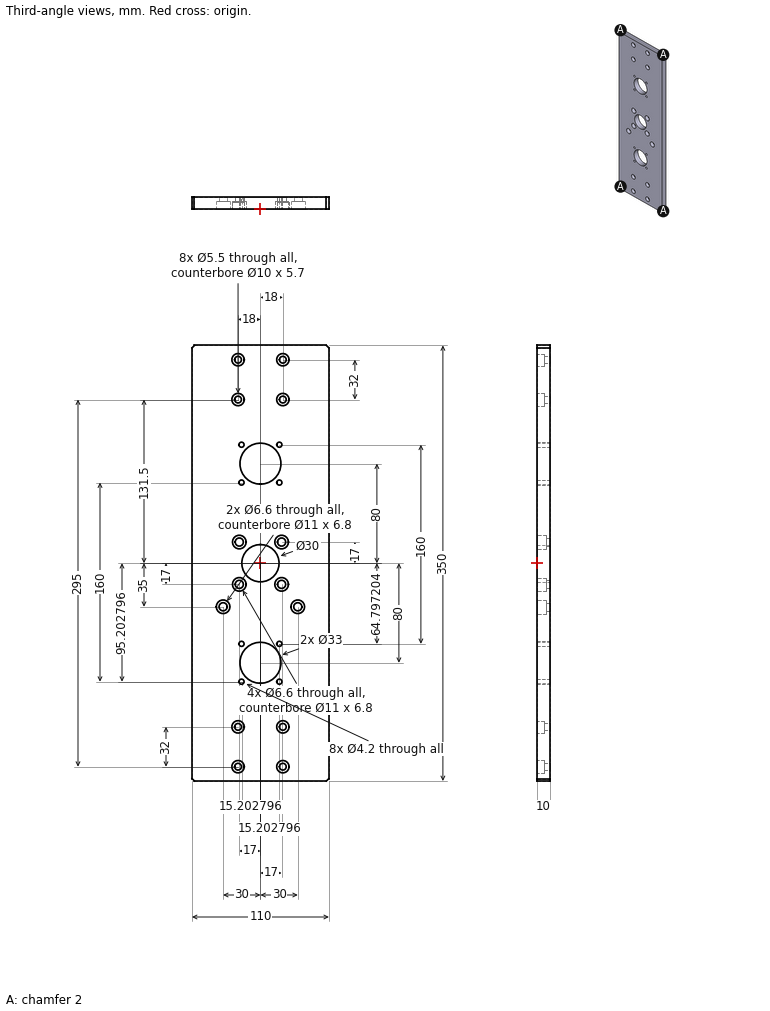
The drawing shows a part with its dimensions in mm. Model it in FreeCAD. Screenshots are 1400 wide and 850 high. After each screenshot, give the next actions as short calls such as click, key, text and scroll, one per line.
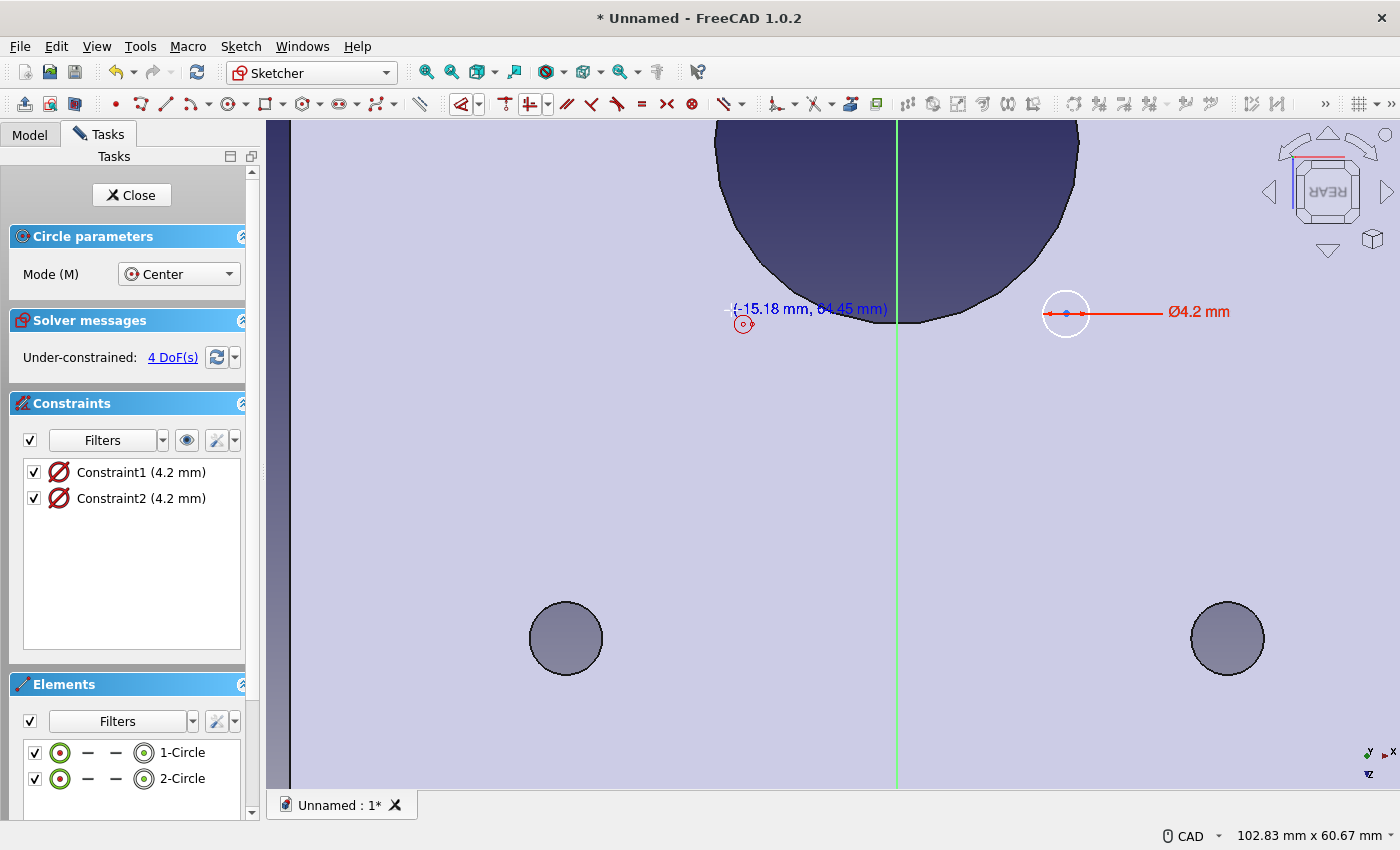
scroll(731, 310, down, 8)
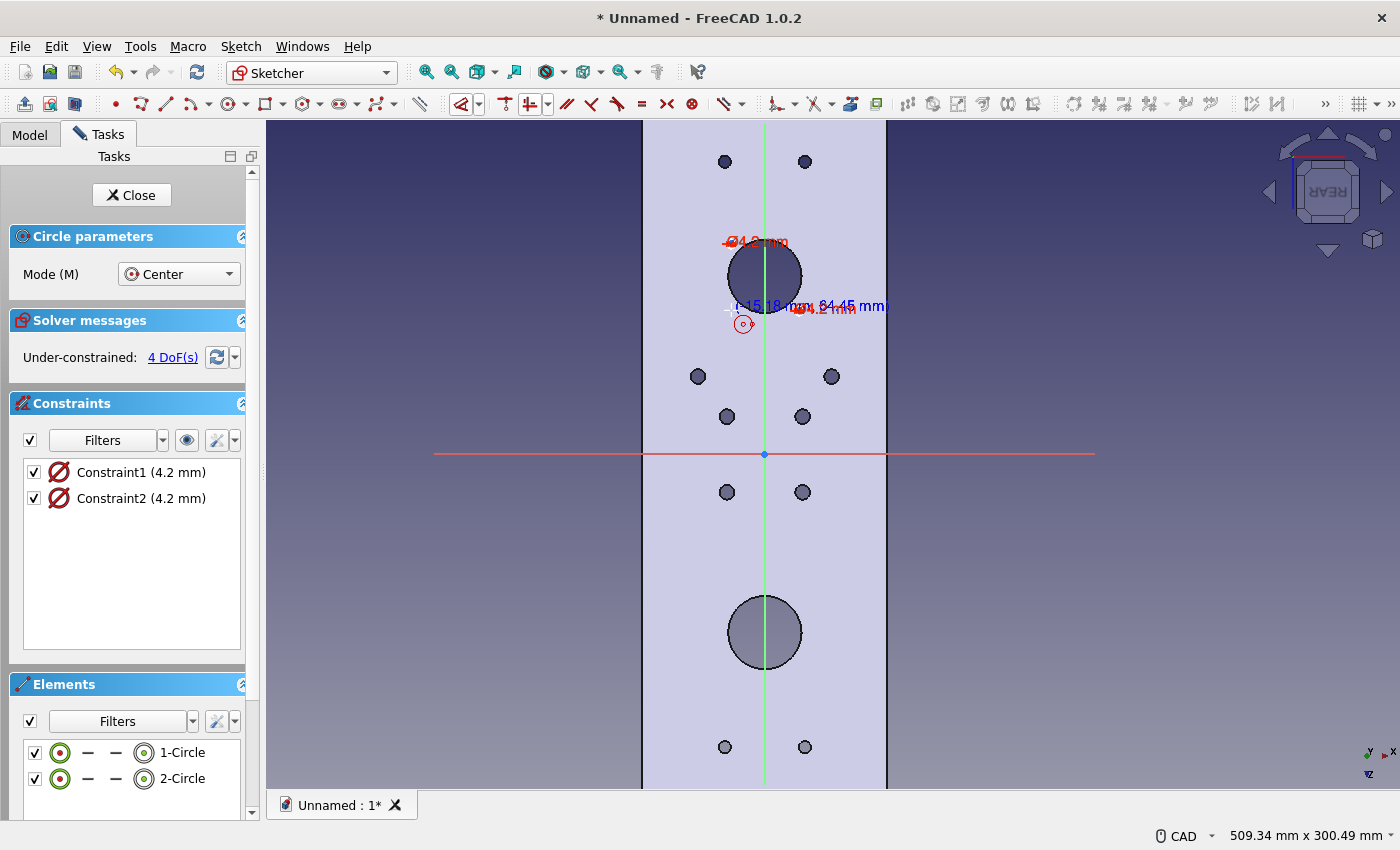
click(731, 310)
move(734, 307)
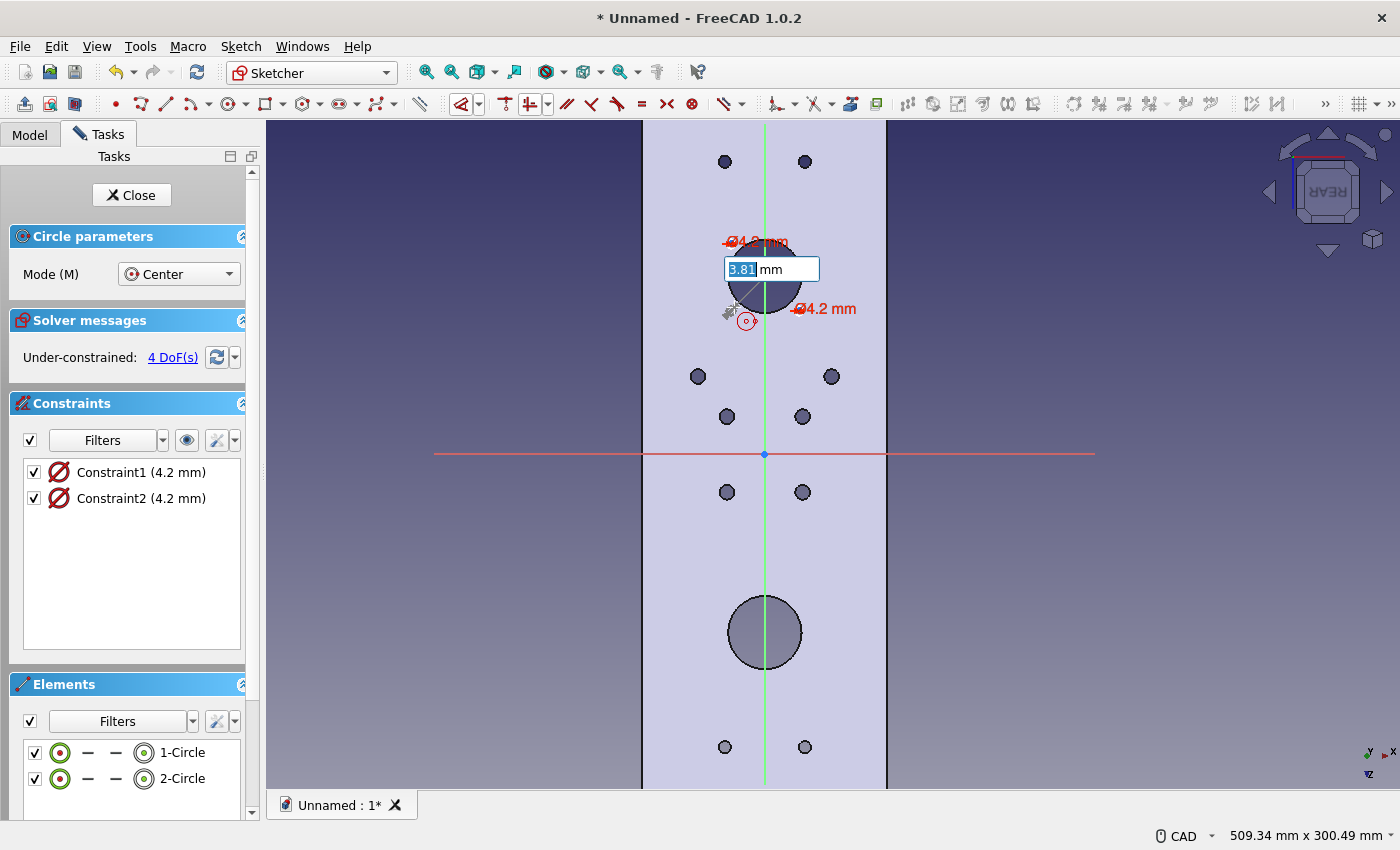
text(4.2)
key(Return)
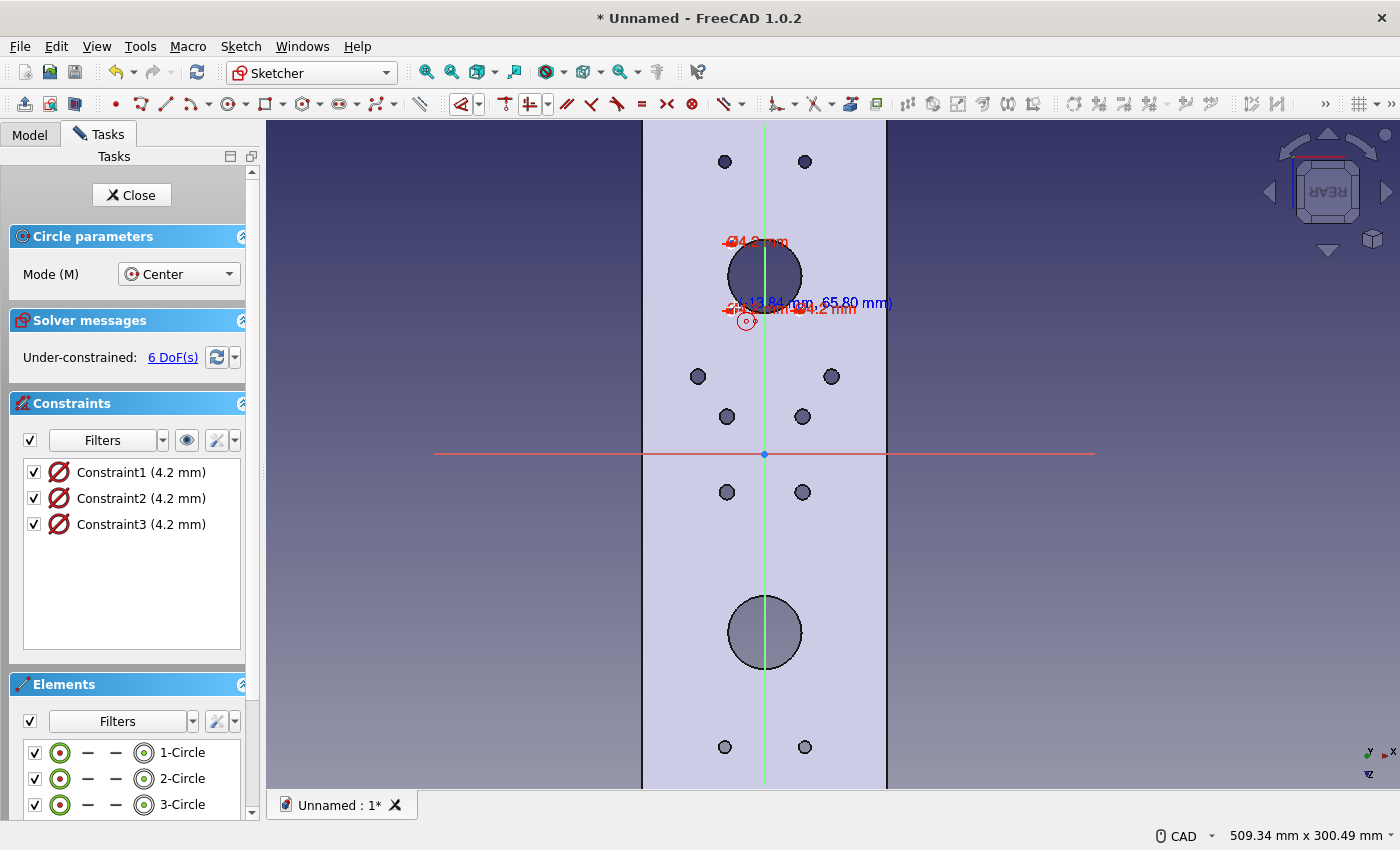
scroll(799, 243, up, 8)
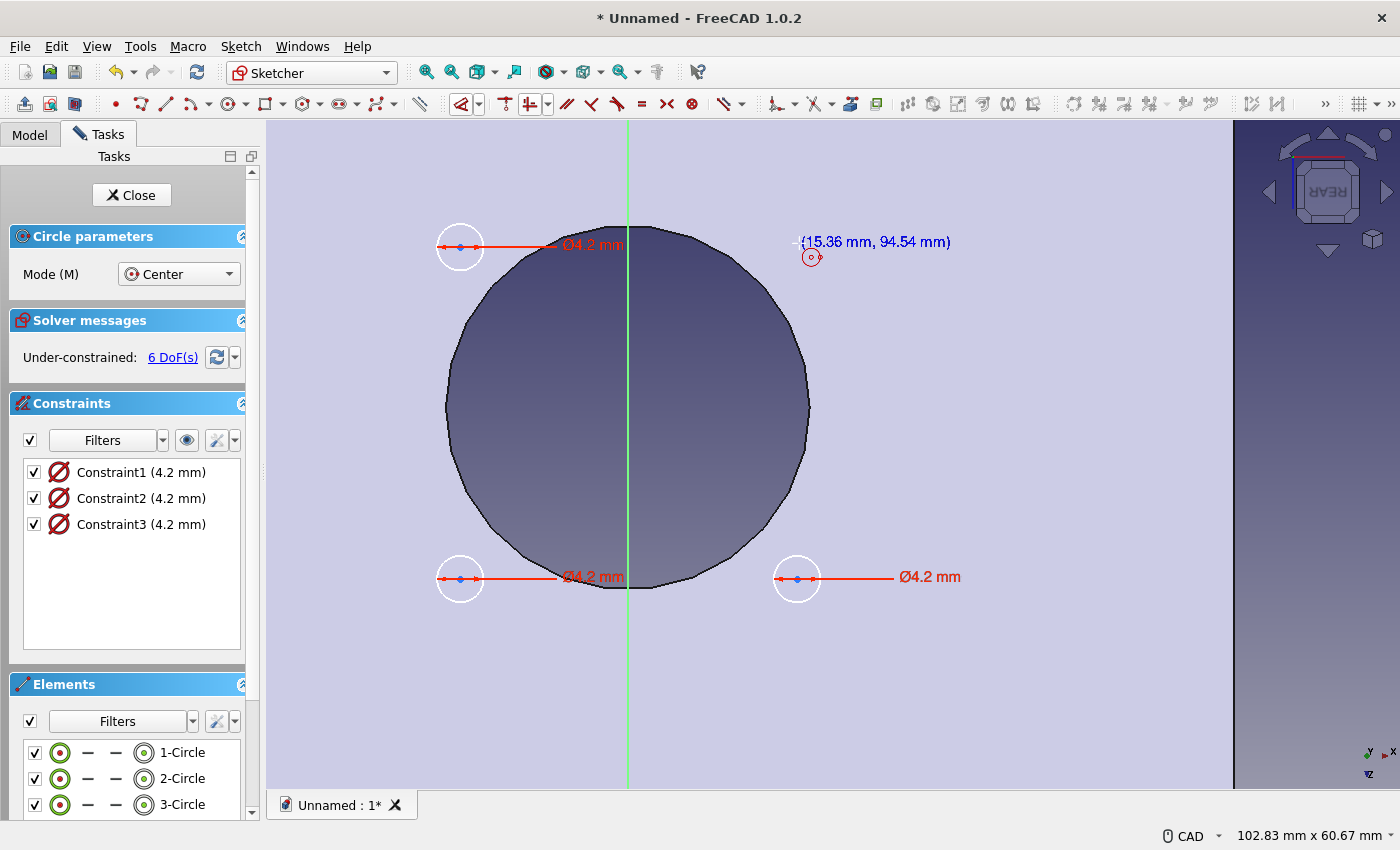
scroll(799, 243, down, 8)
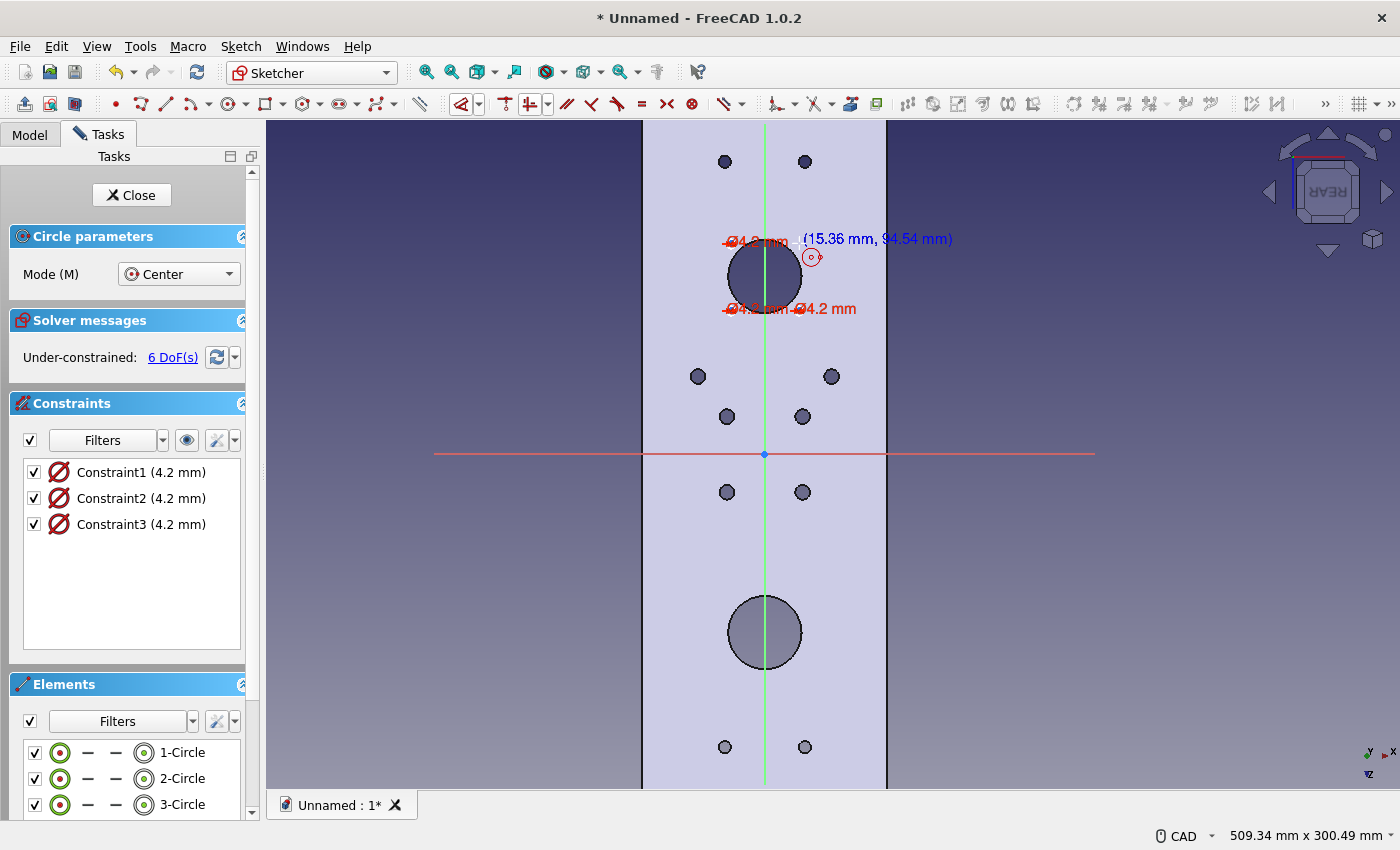
click(799, 243)
move(802, 239)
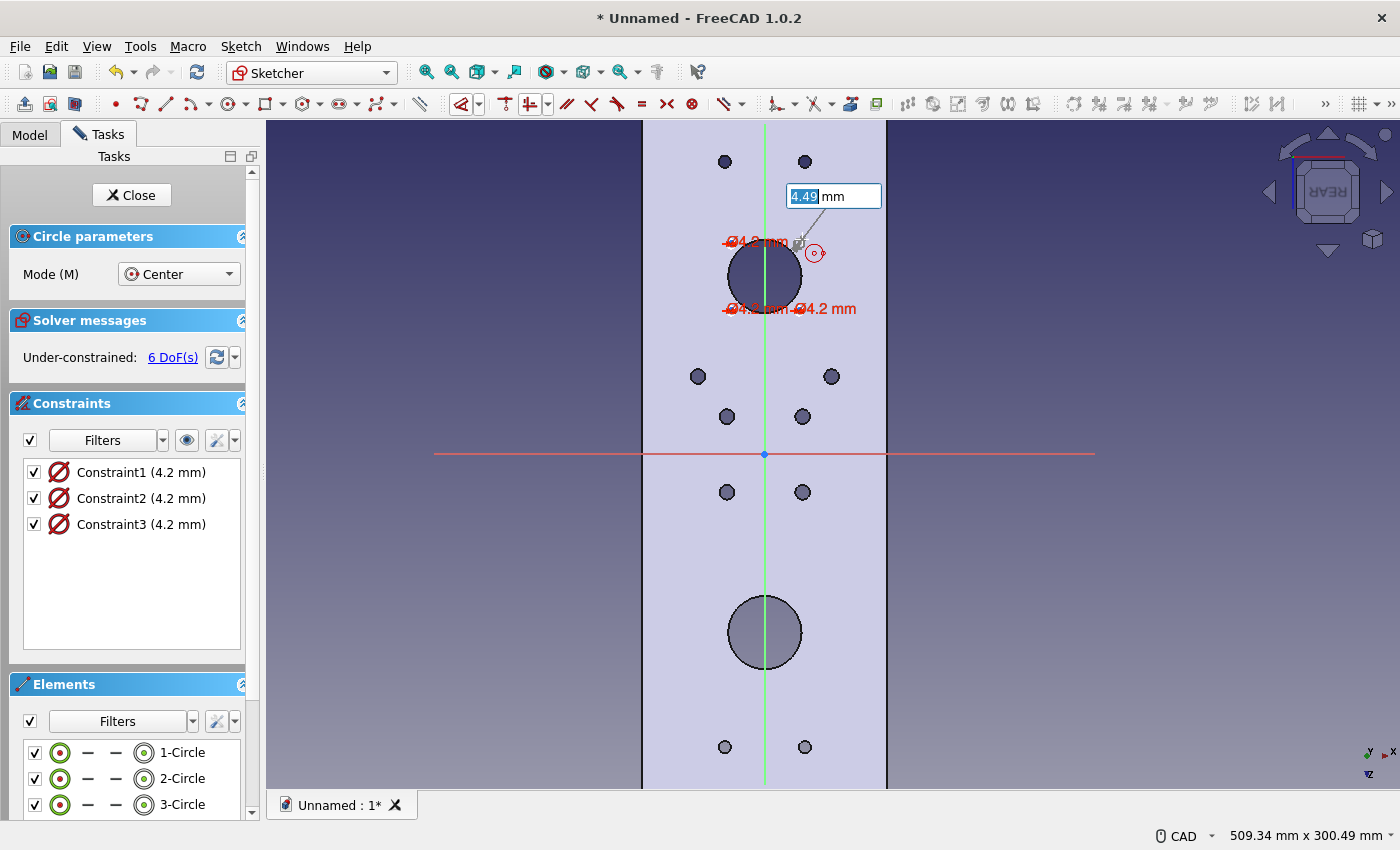
text(4.2)
key(Return)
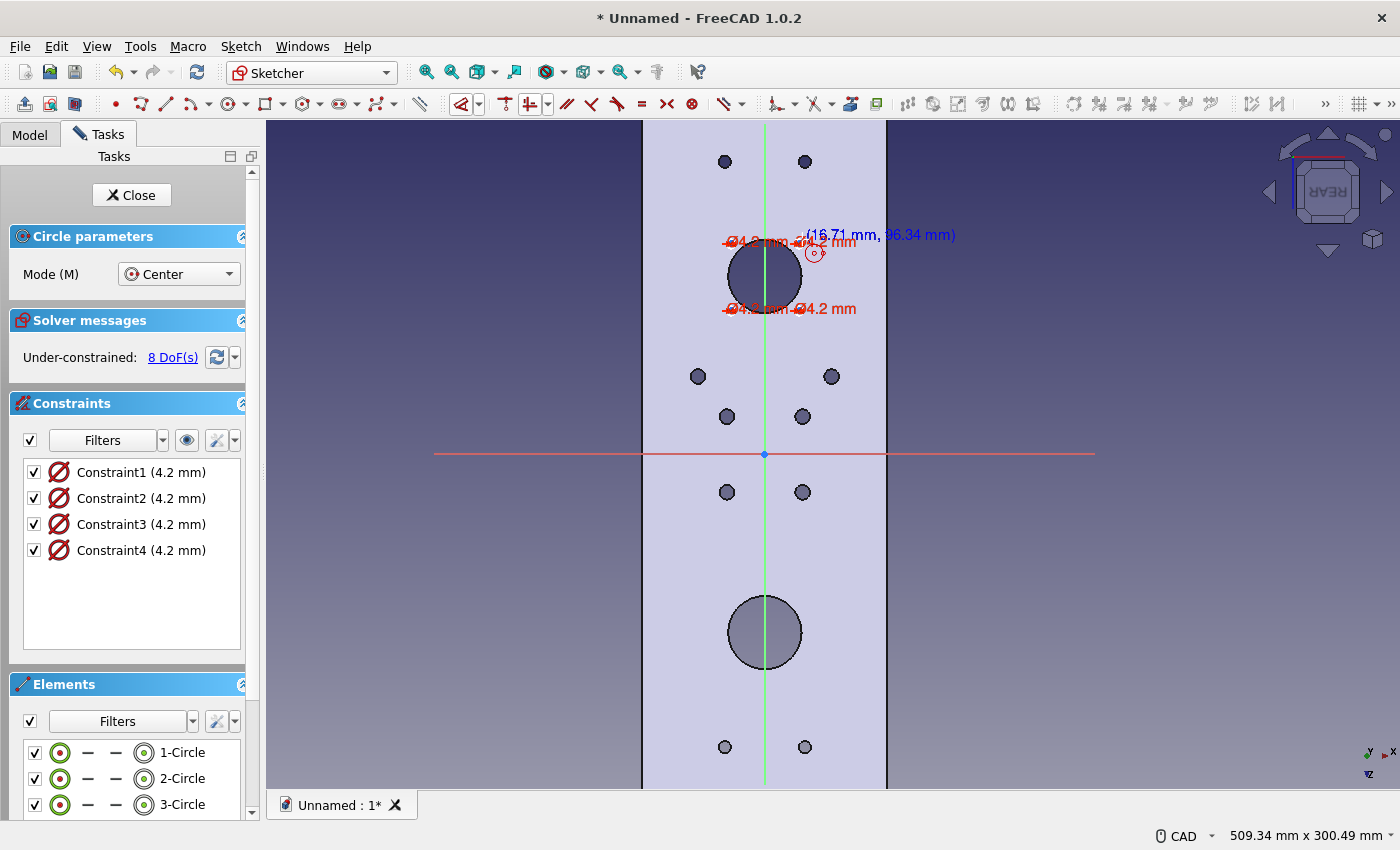
scroll(731, 599, up, 8)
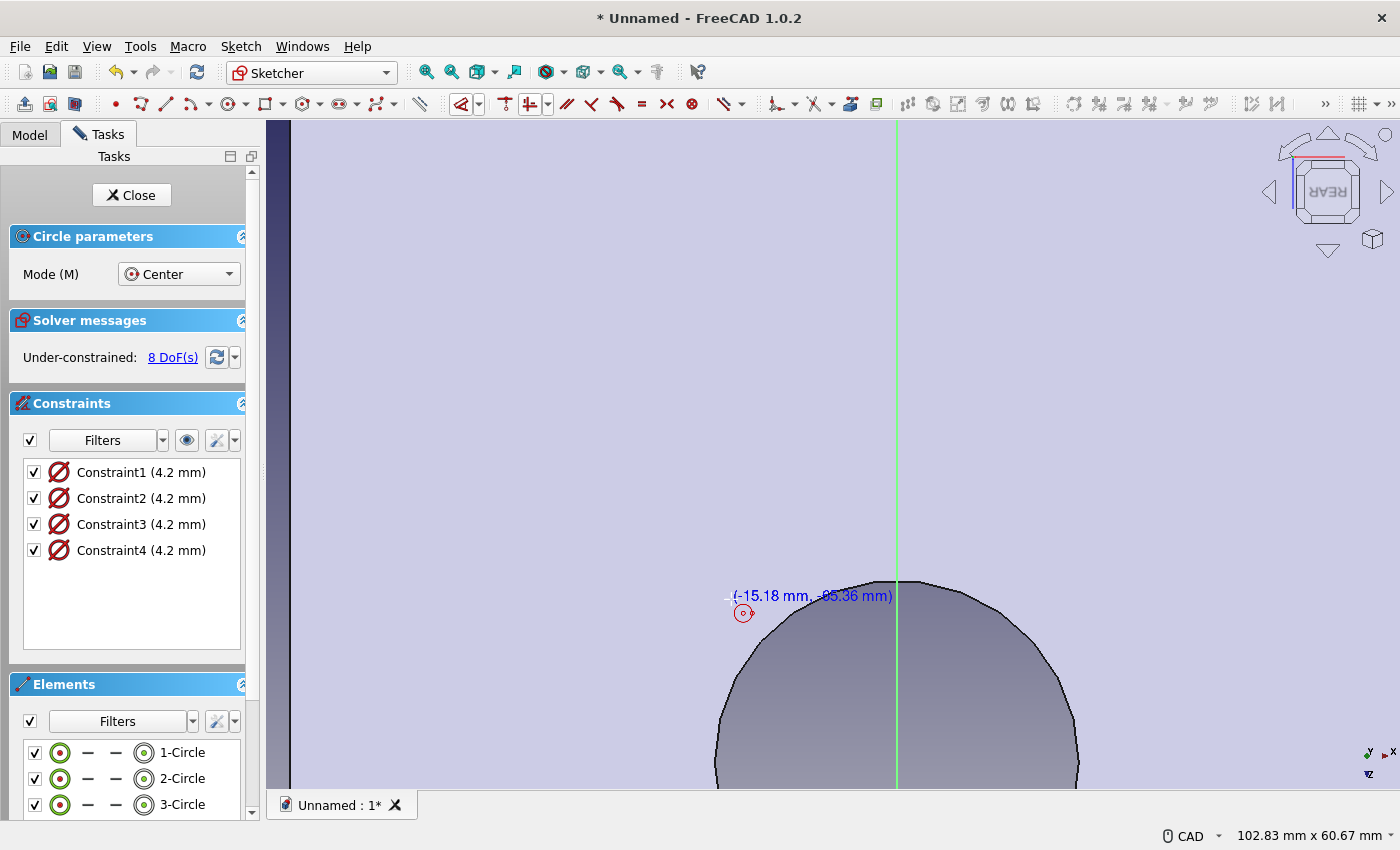
scroll(731, 600, down, 8)